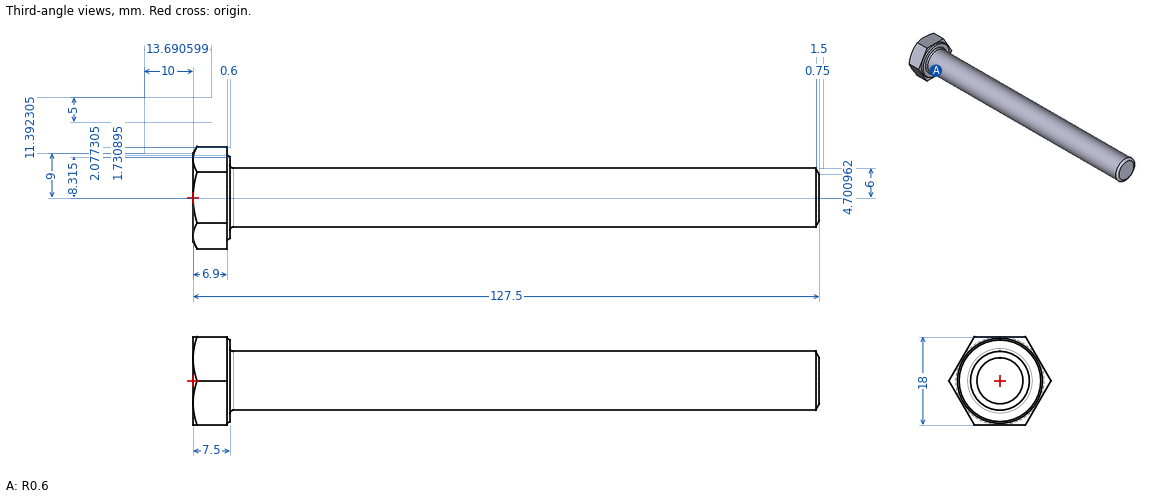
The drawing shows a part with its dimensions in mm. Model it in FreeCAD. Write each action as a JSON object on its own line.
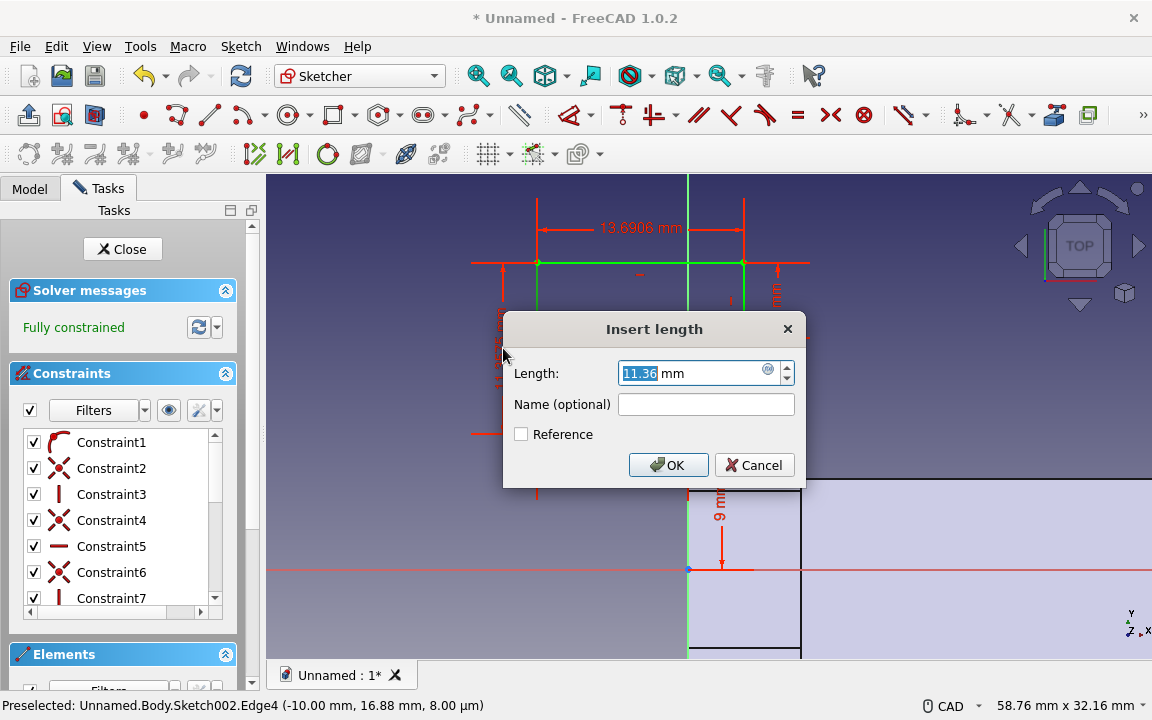
{"action": "type", "text": "11.392305"}
{"action": "key", "text": "Return"}
{"action": "key", "text": "Escape"}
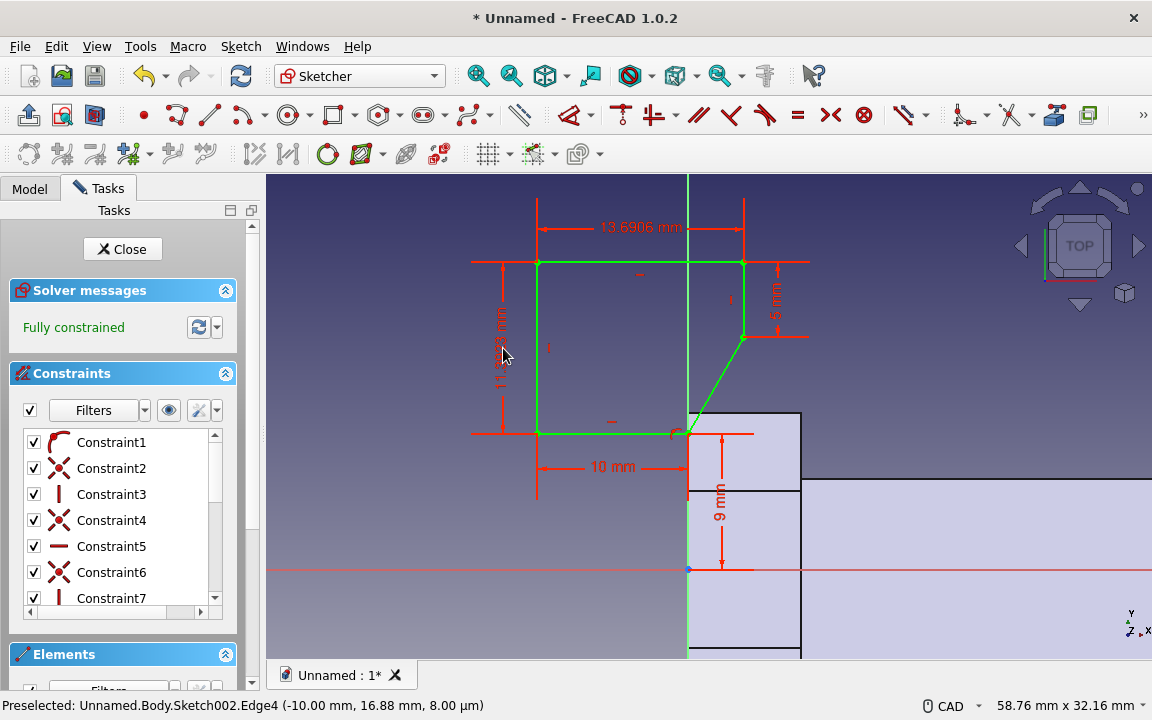
{"action": "left_click", "coordinate": [123, 249]}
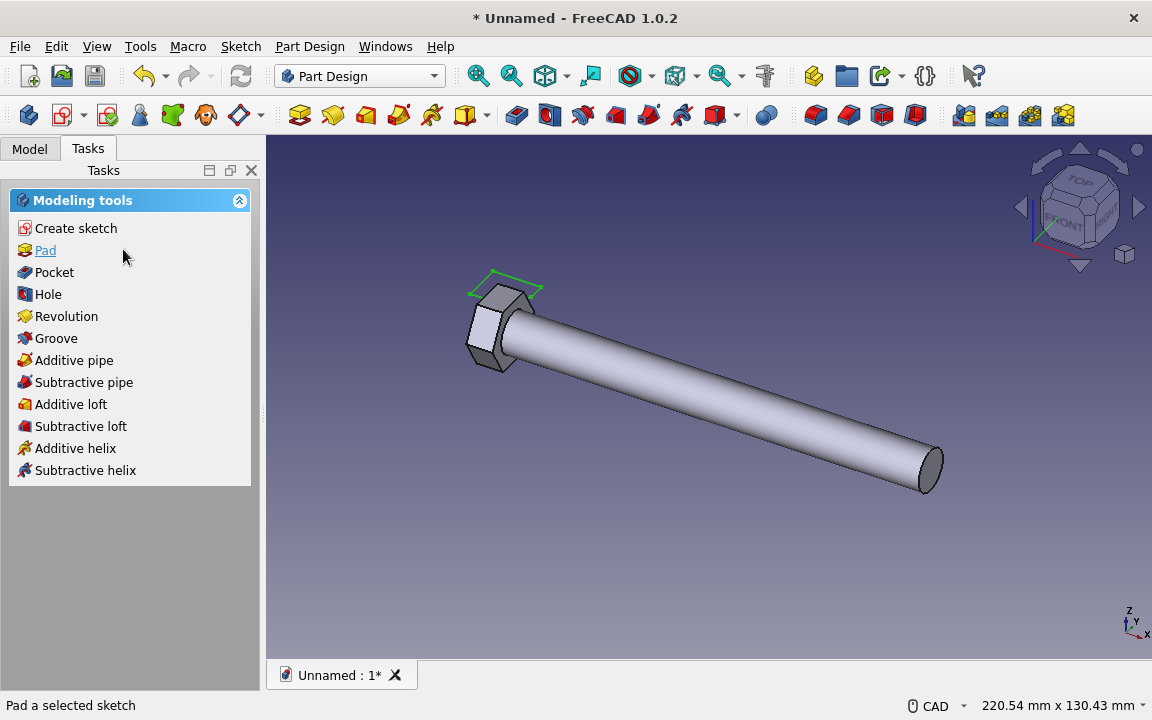
{"action": "left_click", "coordinate": [583, 116]}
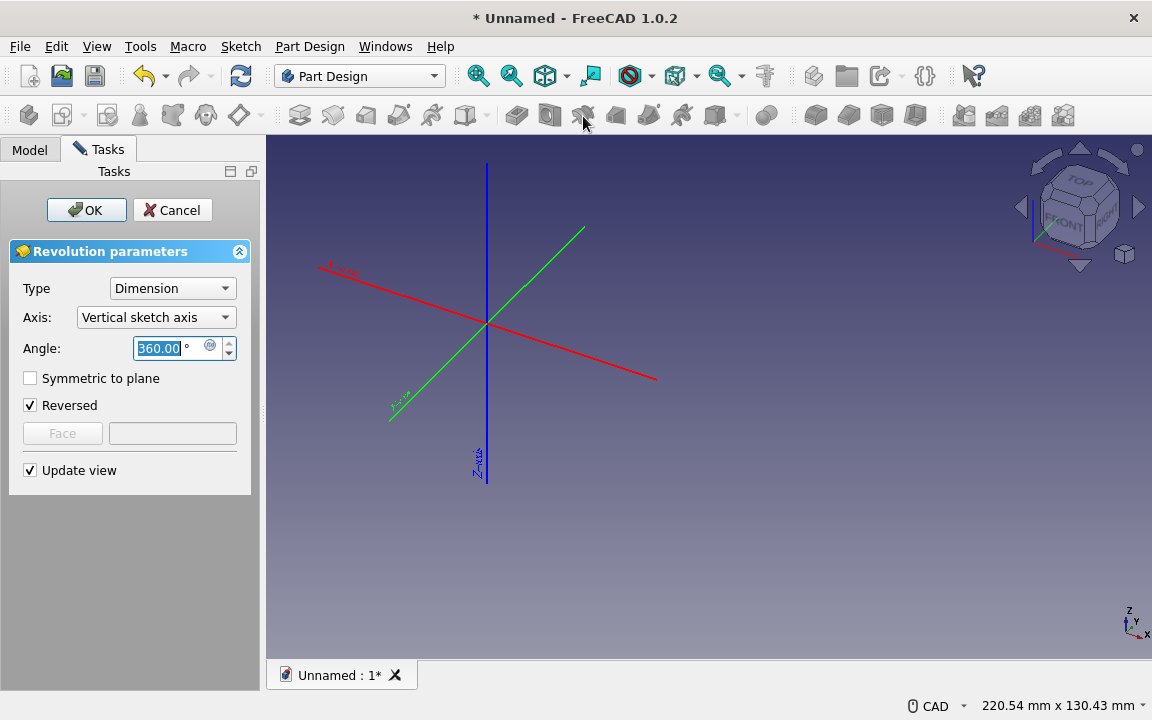
{"action": "left_click", "coordinate": [157, 318]}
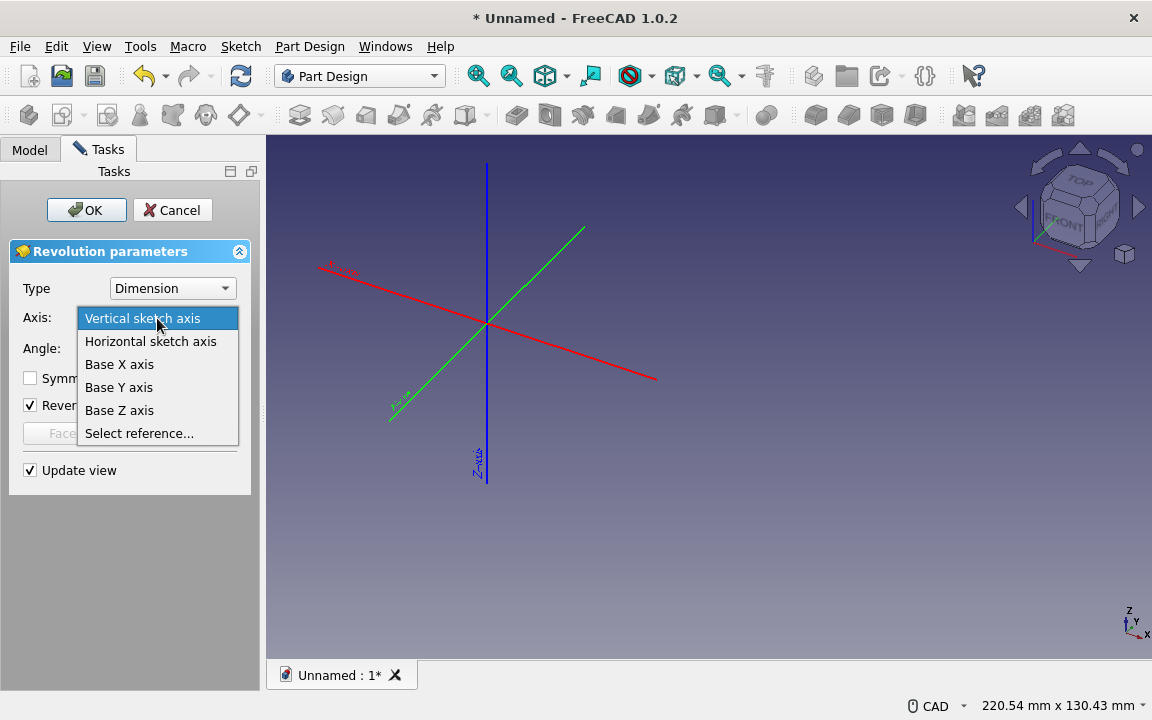
{"action": "left_click", "coordinate": [156, 342]}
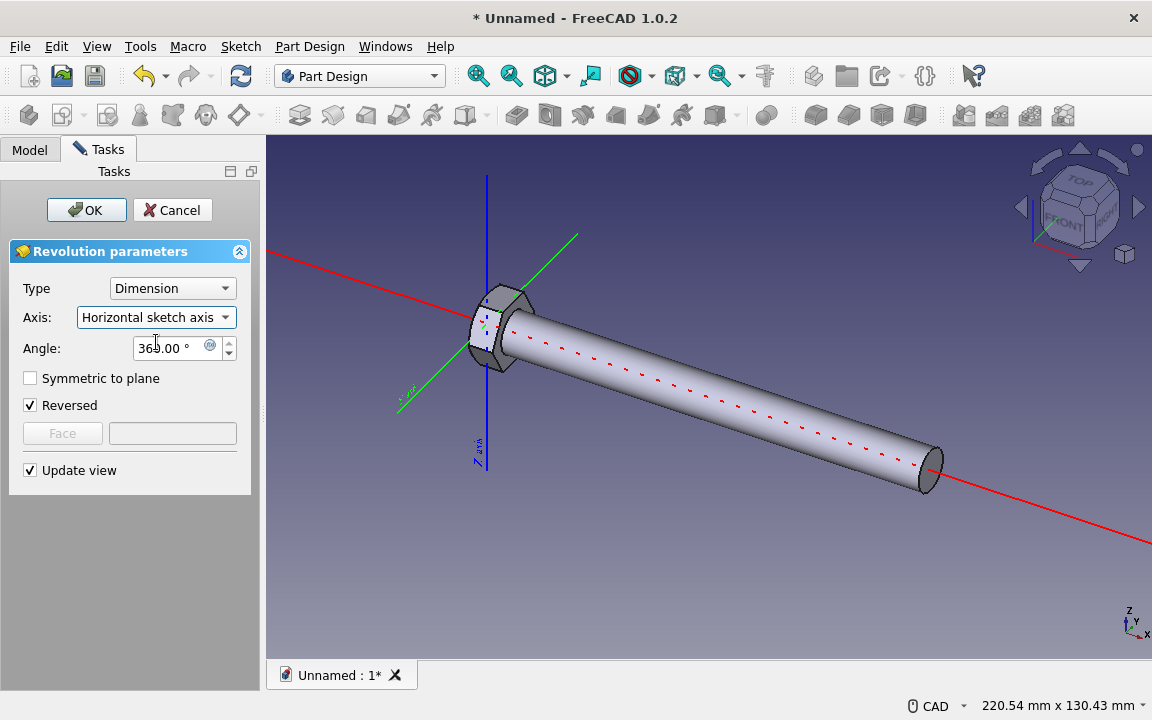
{"action": "left_click", "coordinate": [87, 210]}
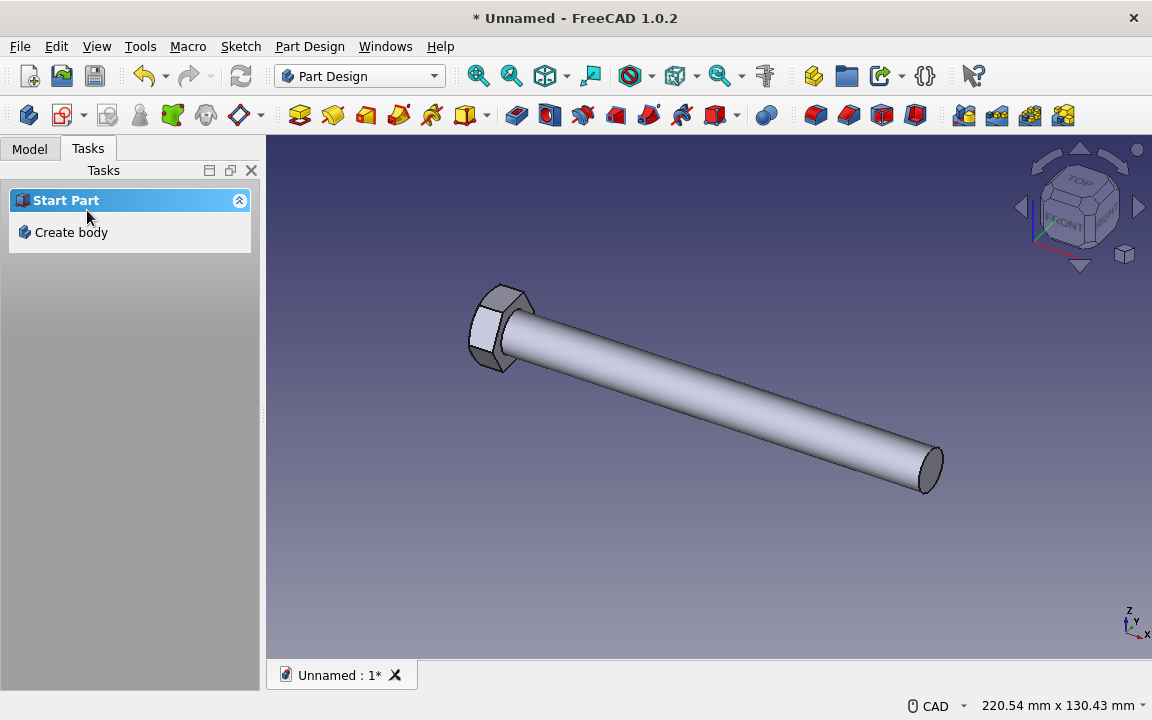
{"action": "left_click", "coordinate": [62, 116]}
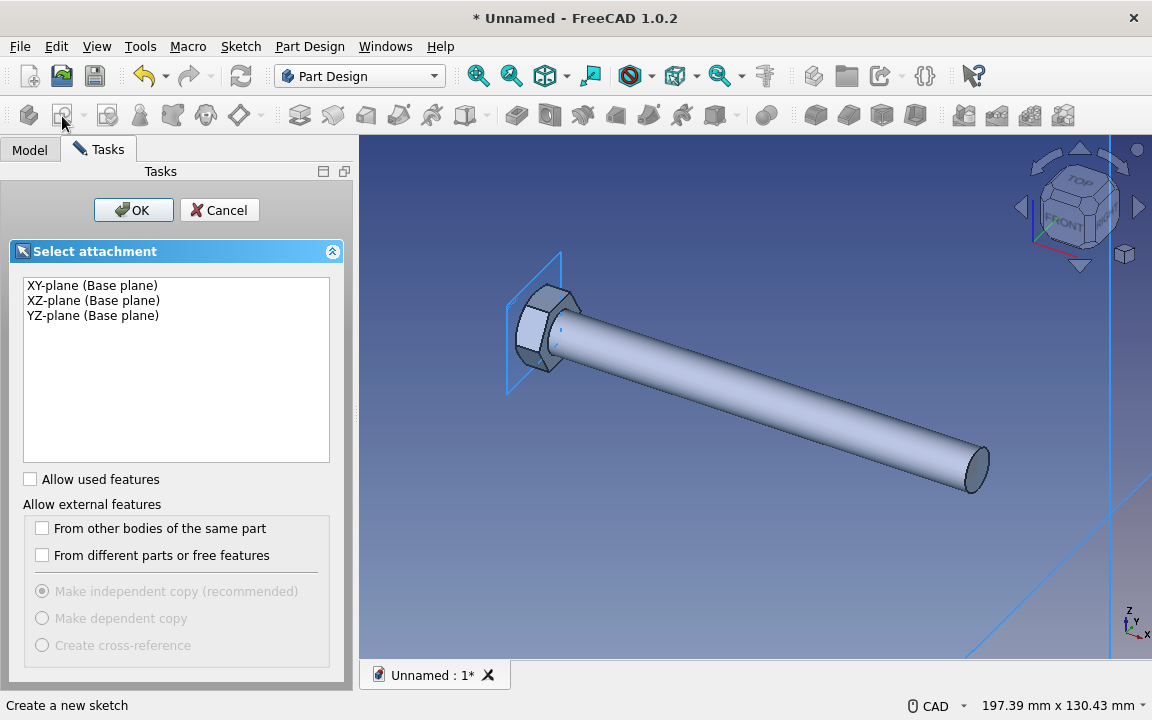
{"action": "left_click", "coordinate": [84, 286]}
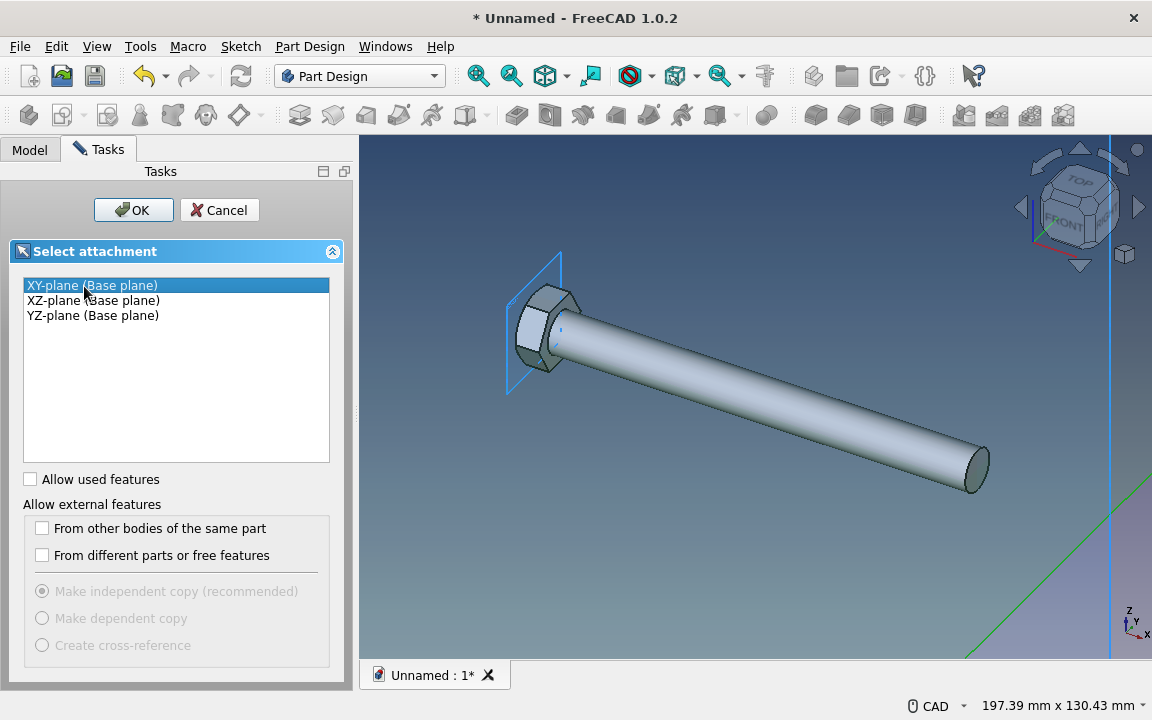
{"action": "left_click", "coordinate": [134, 210]}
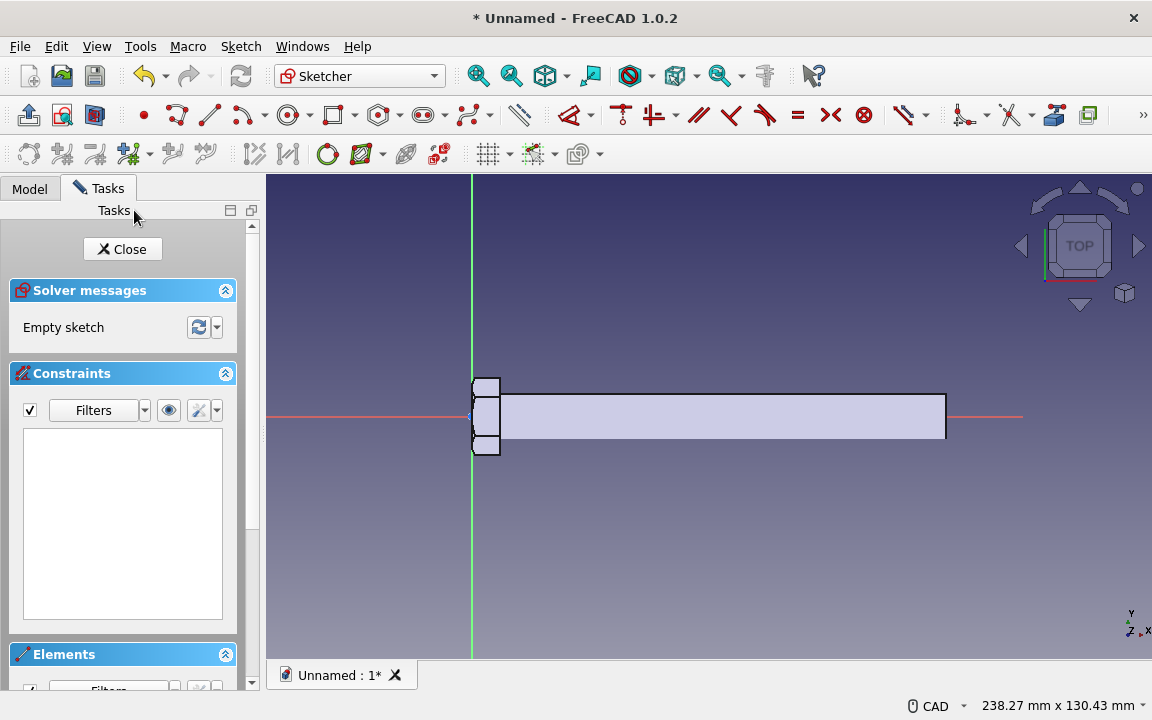
{"action": "left_click", "coordinate": [95, 116]}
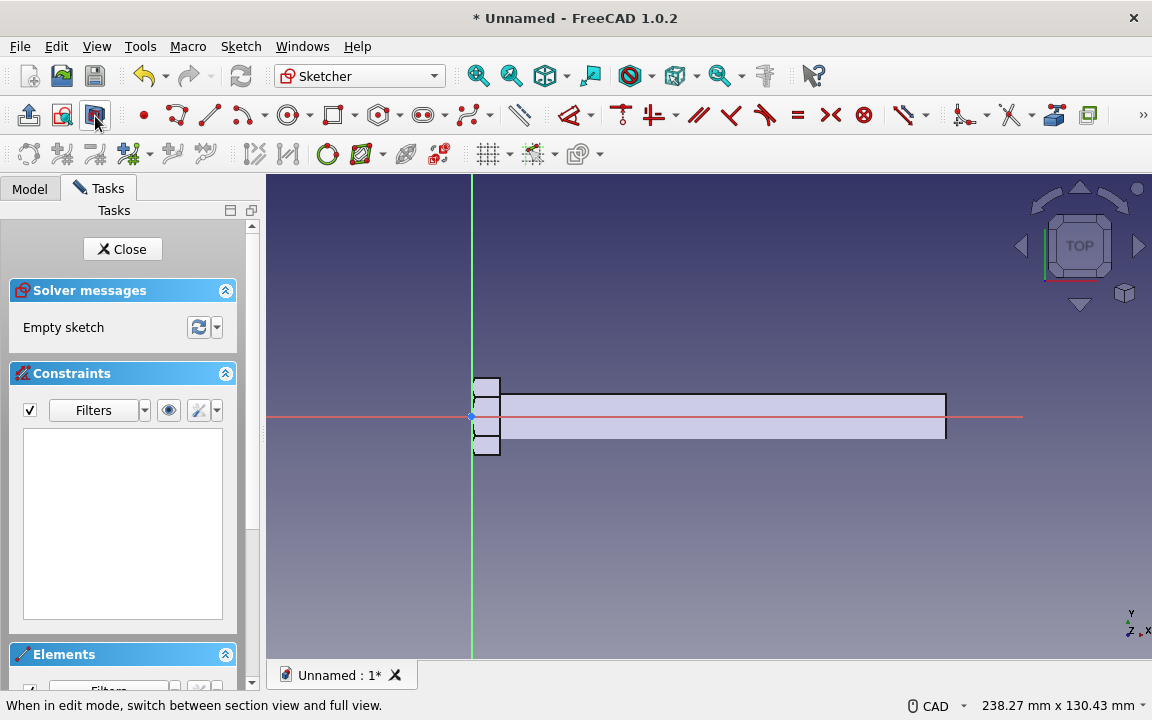
{"action": "scroll", "coordinate": [491, 380], "scroll_direction": "up", "scroll_amount": 15}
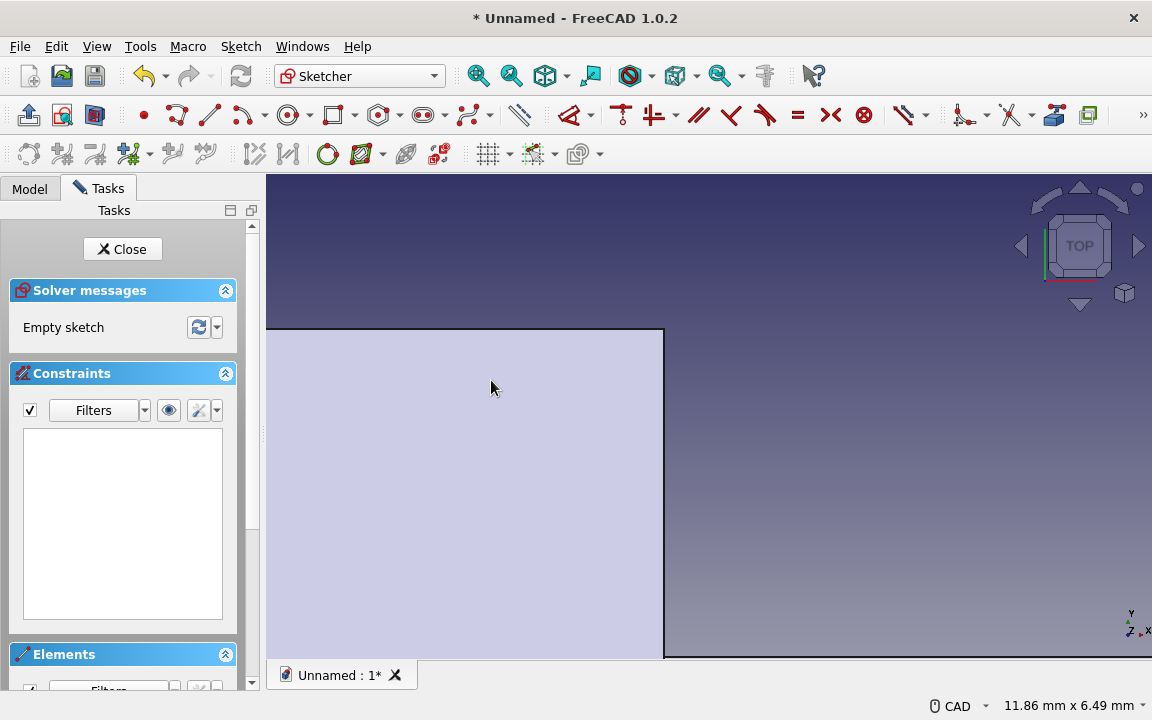
{"action": "scroll", "coordinate": [642, 394], "scroll_direction": "up", "scroll_amount": 3}